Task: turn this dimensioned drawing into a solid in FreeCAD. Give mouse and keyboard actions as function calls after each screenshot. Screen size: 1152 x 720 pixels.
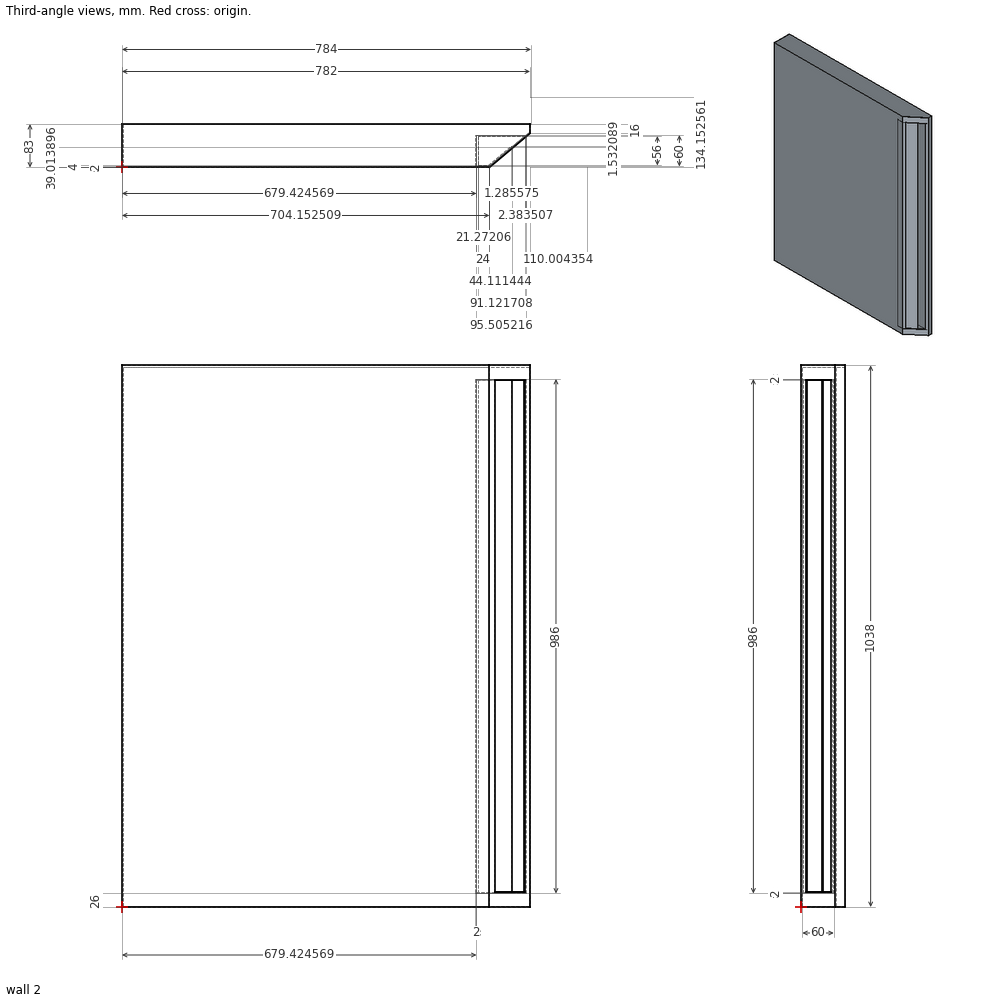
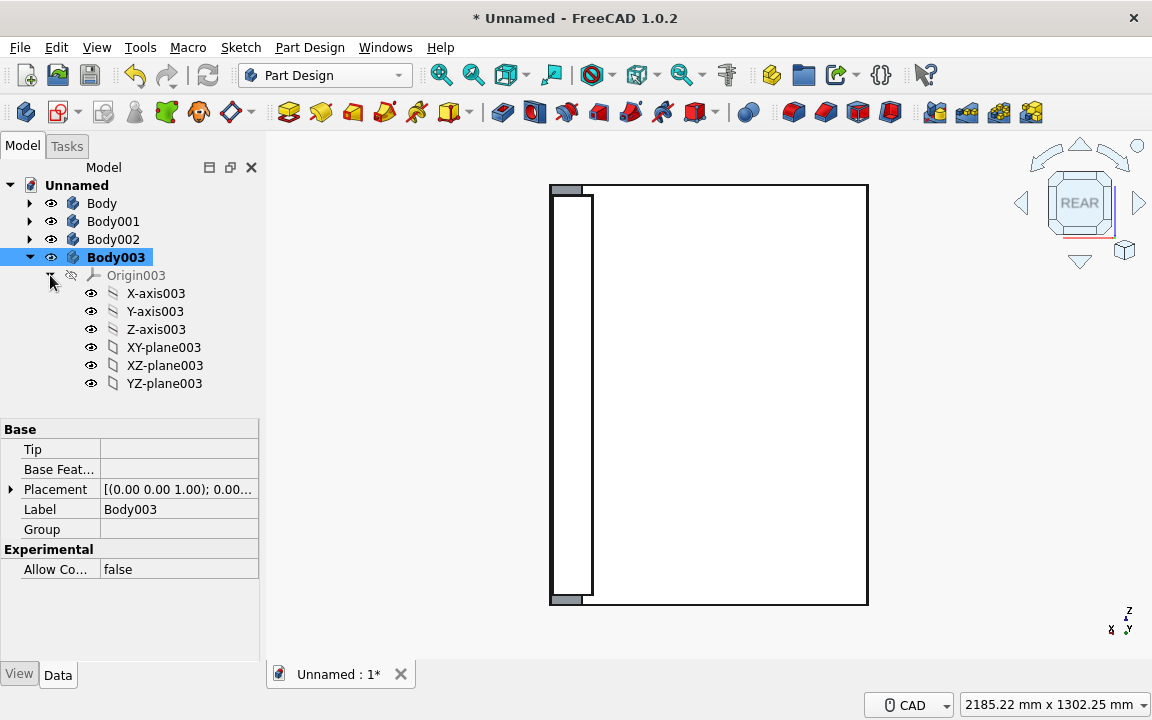
click(136, 347)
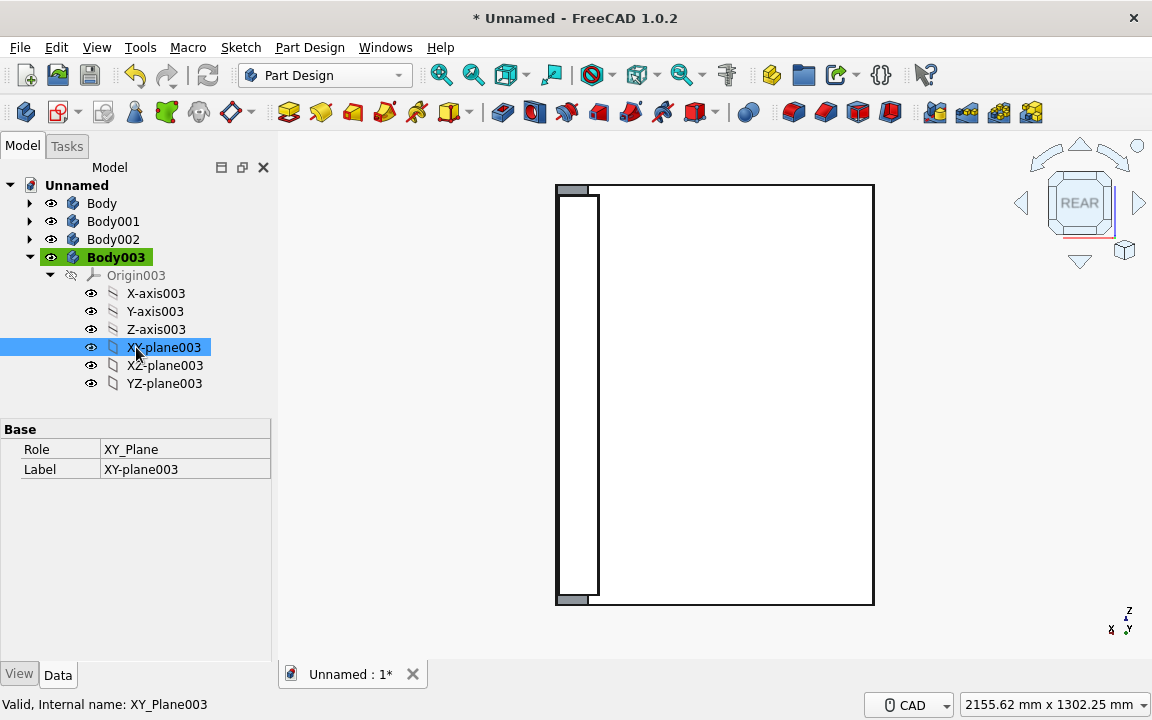
click(232, 112)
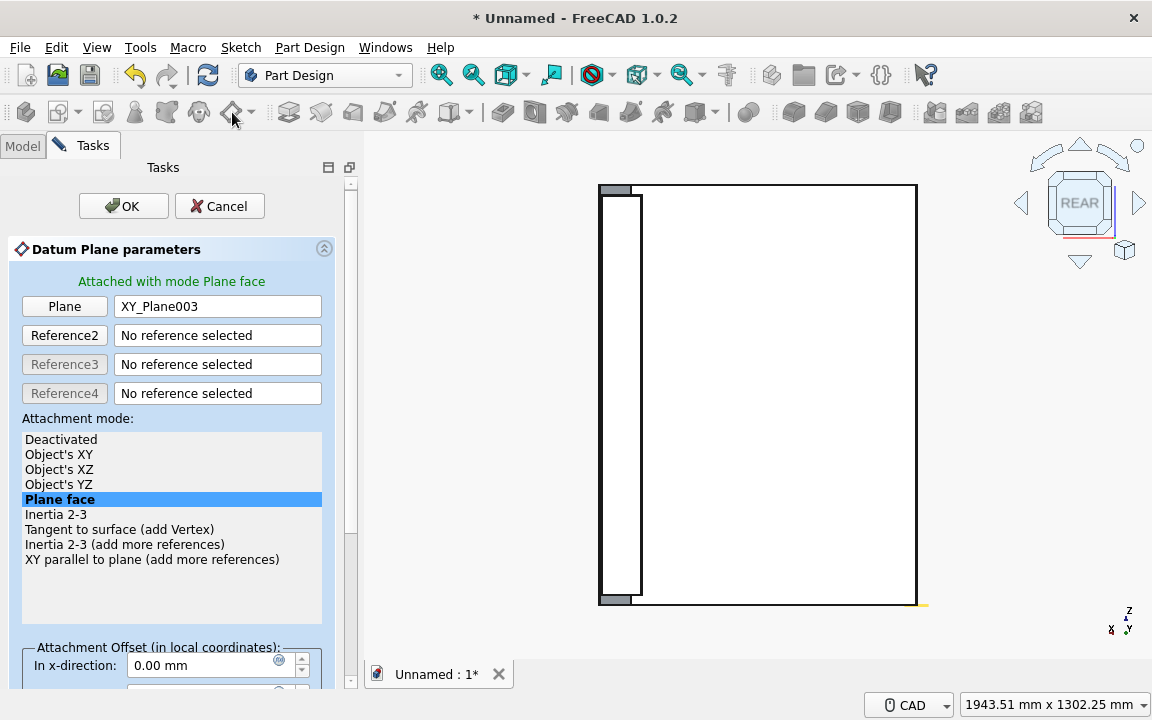
scroll(351, 432, down, 2)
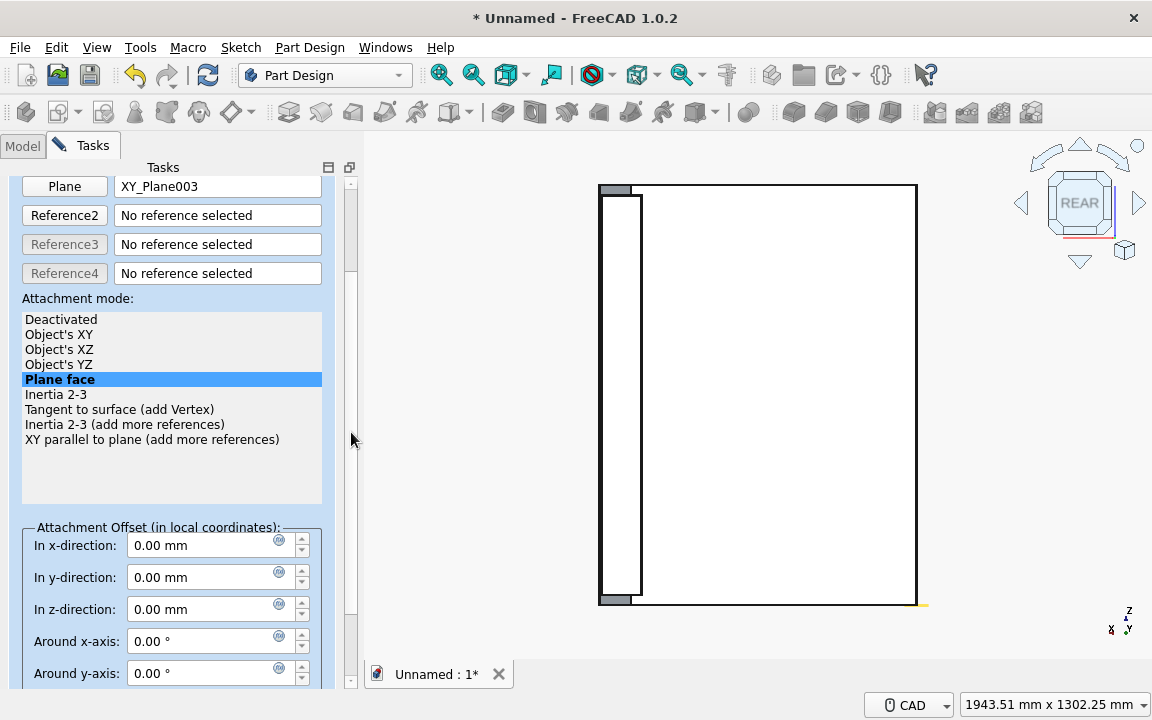
triple_click(210, 609)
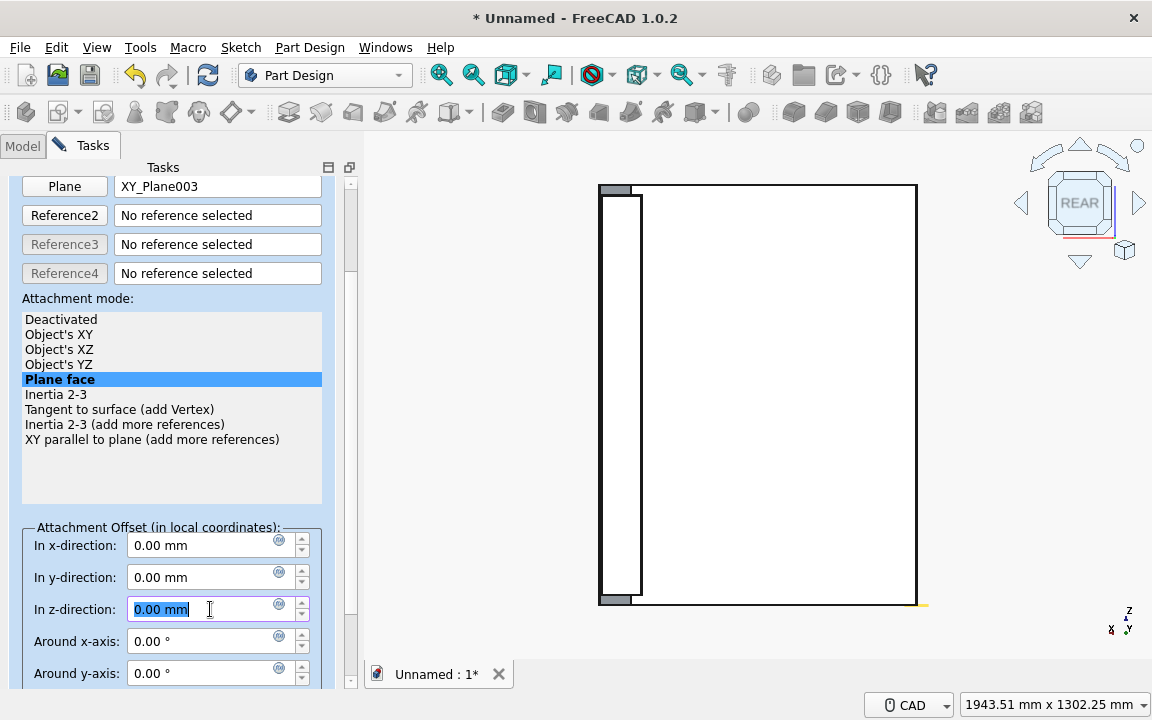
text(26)
key(Tab)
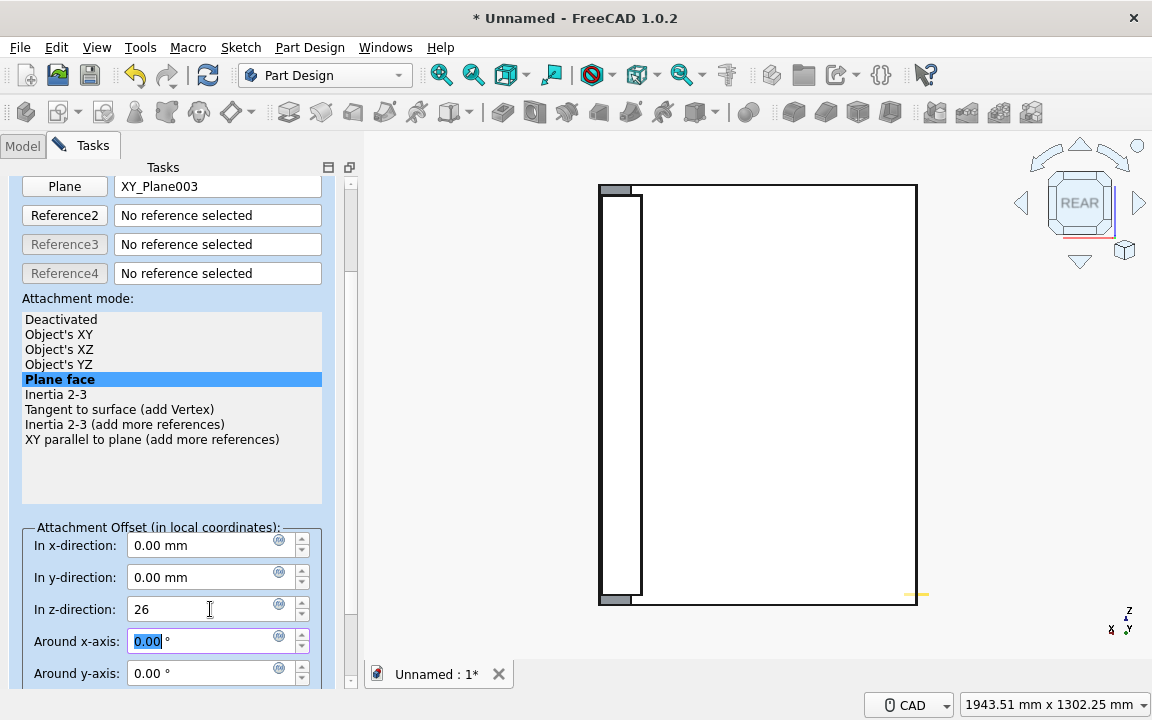
scroll(351, 432, up, 3)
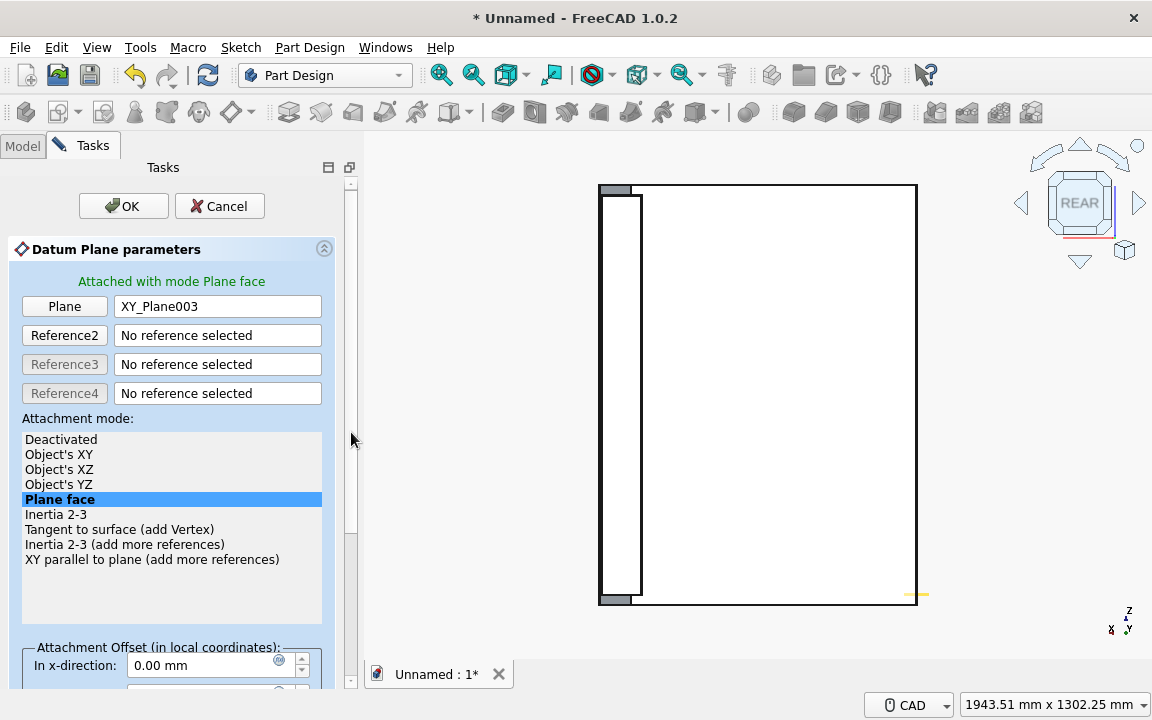
click(124, 206)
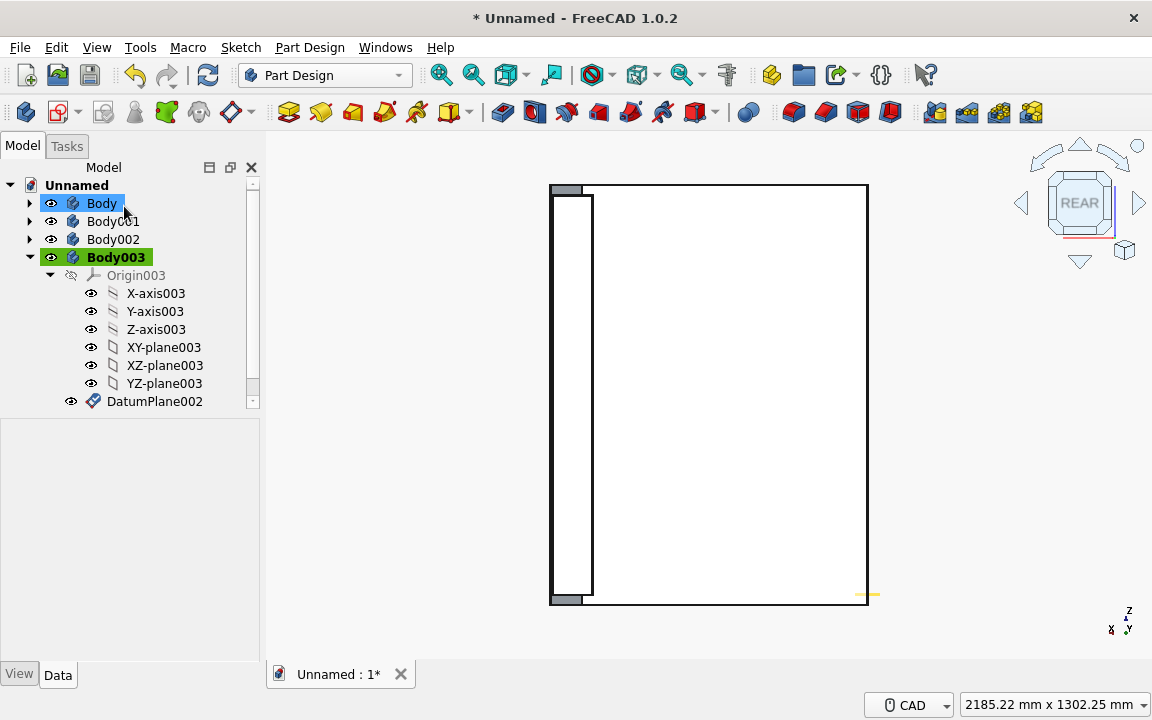
click(116, 401)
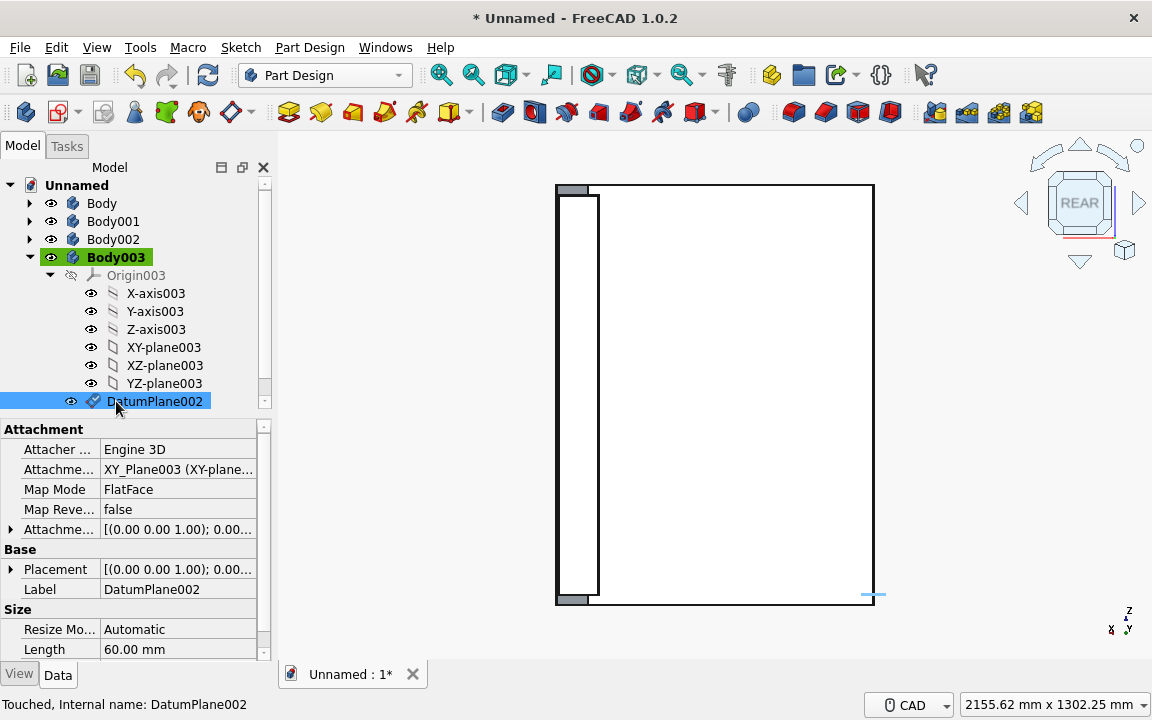
click(58, 112)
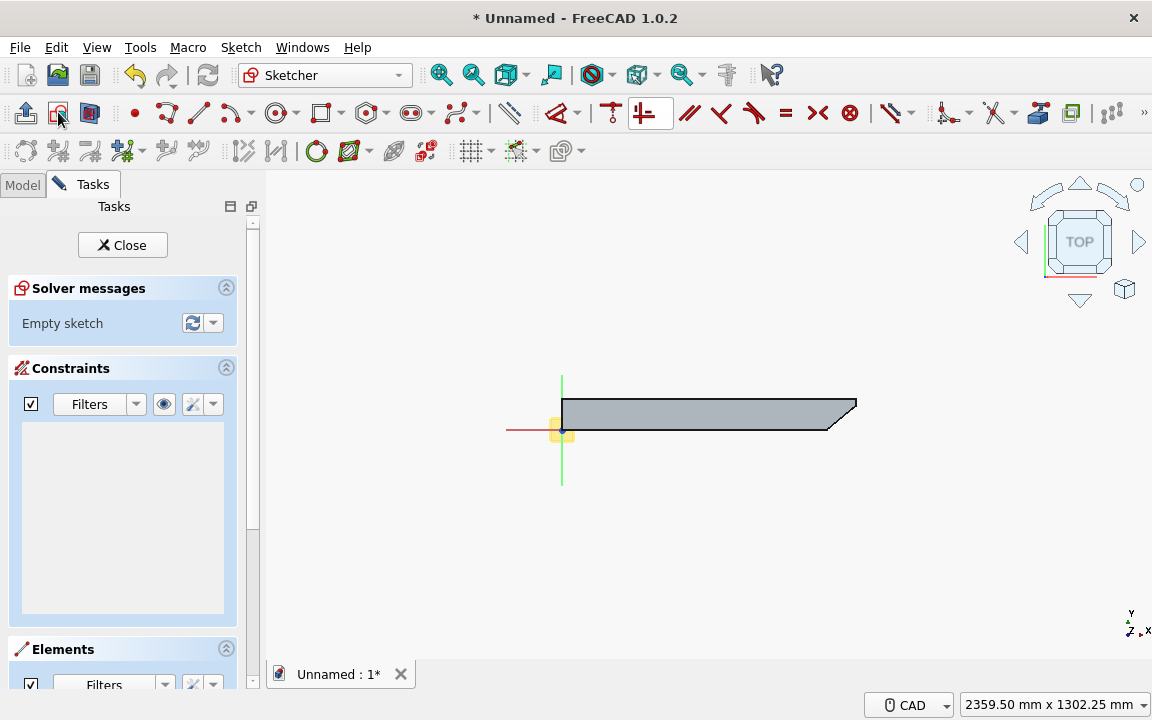
scroll(851, 418, up, 13)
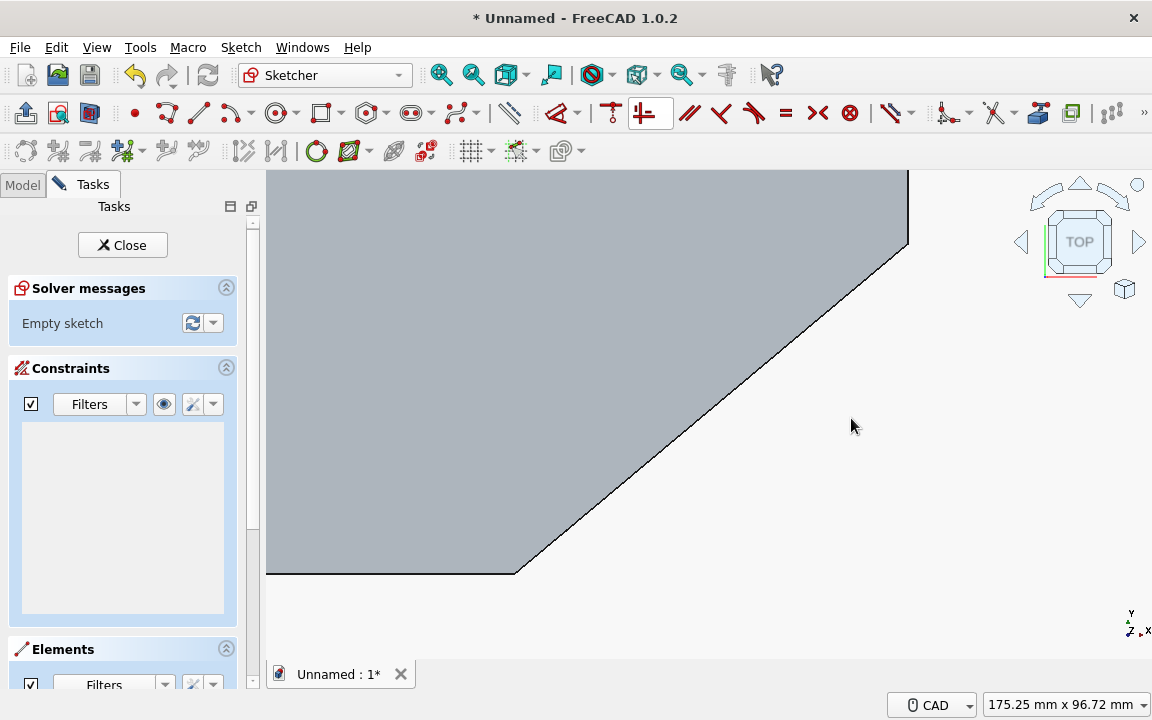
click(168, 114)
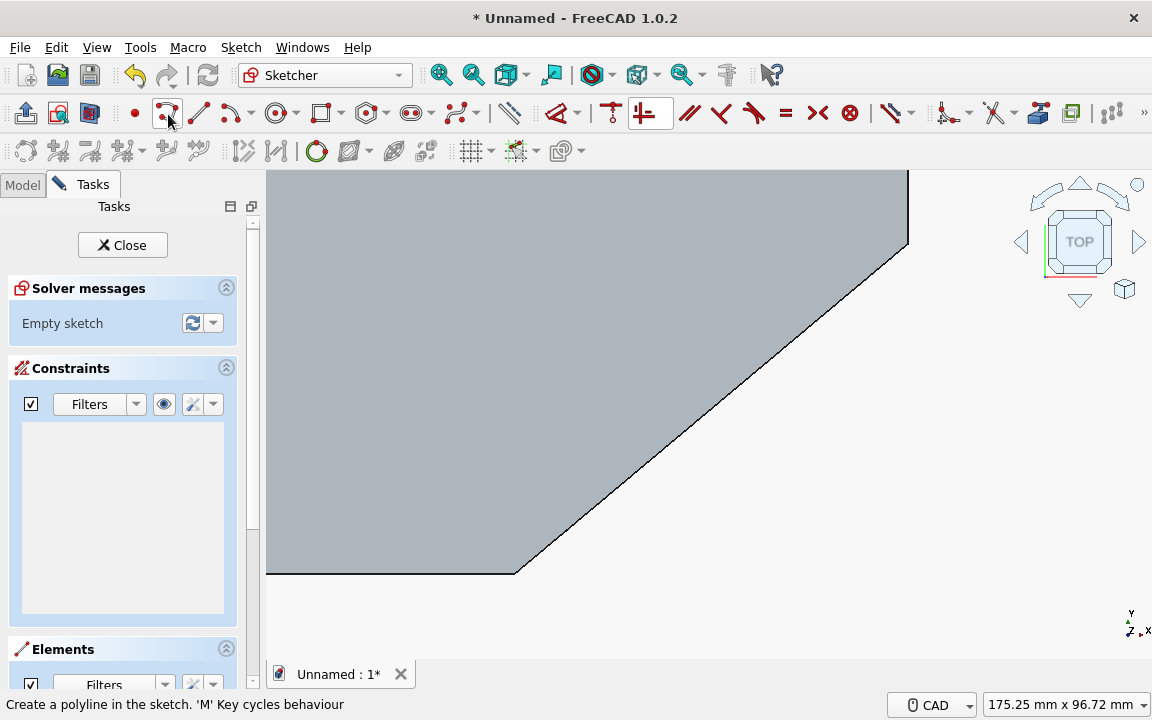
scroll(389, 564, up, 3)